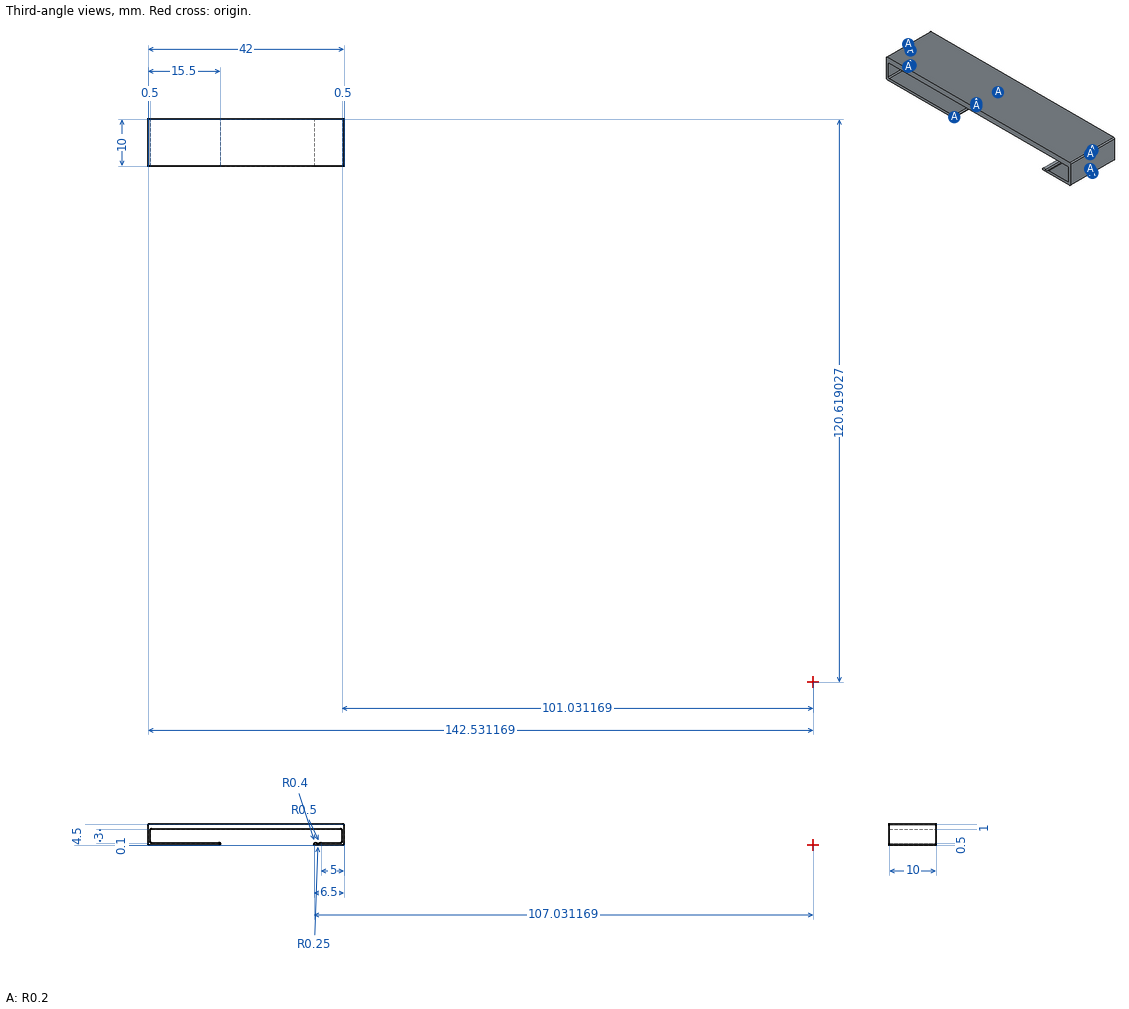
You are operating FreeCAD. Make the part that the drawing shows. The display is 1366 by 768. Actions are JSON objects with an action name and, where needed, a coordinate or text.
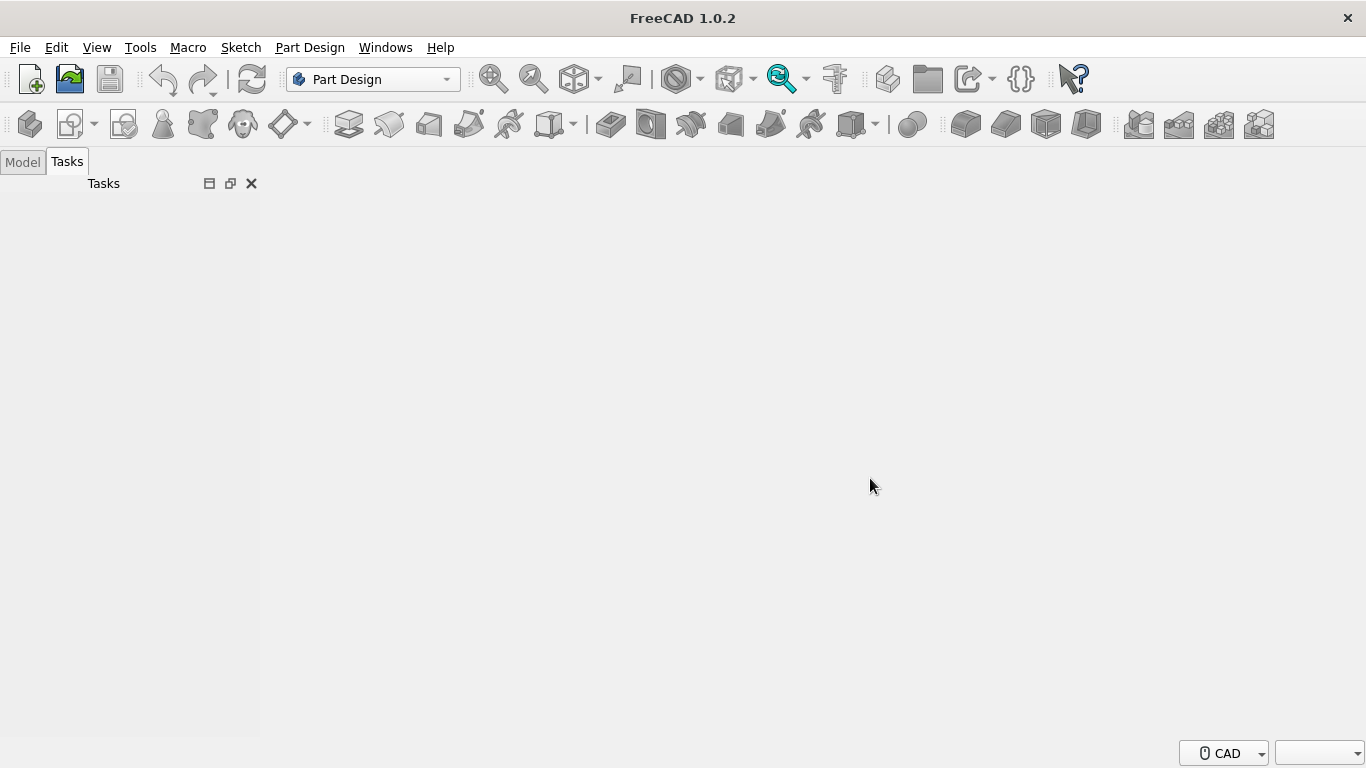
{"action": "left_click", "coordinate": [30, 80]}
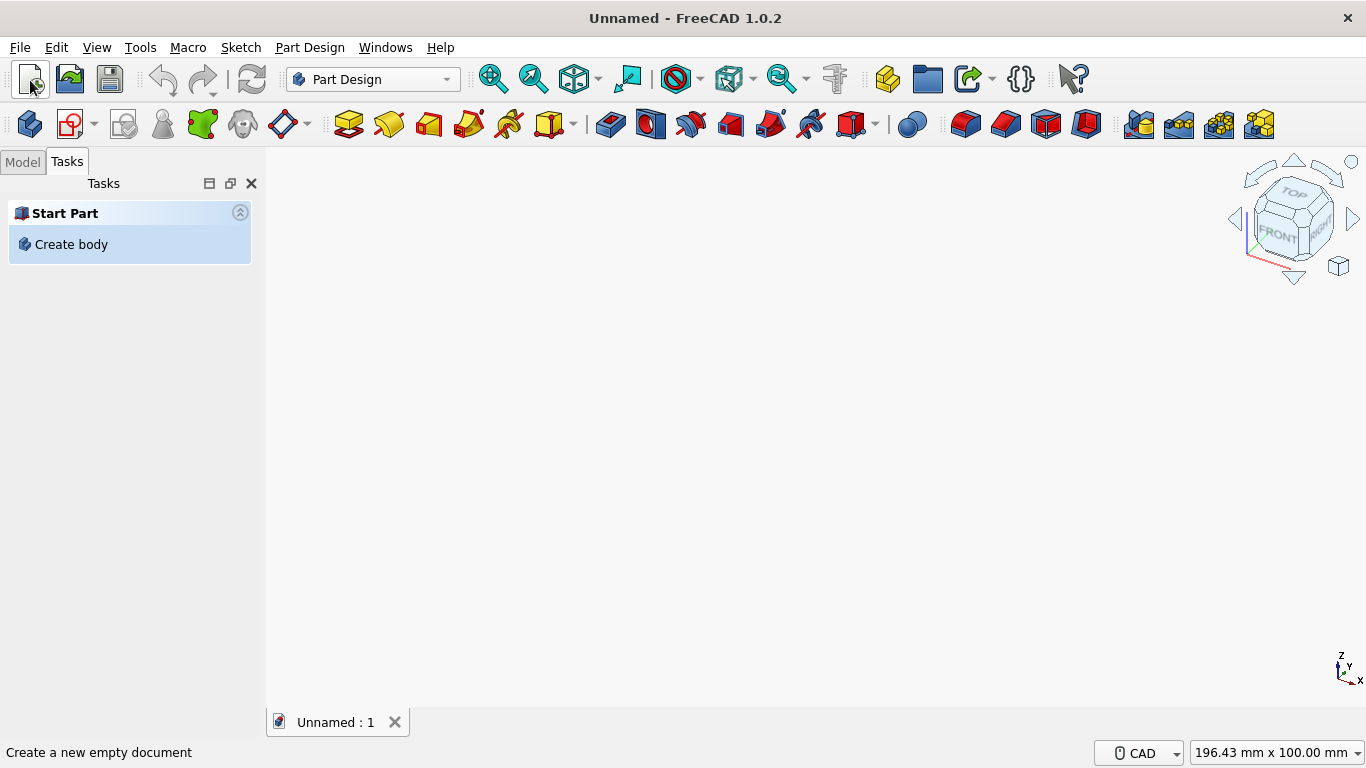
{"action": "left_click", "coordinate": [70, 124]}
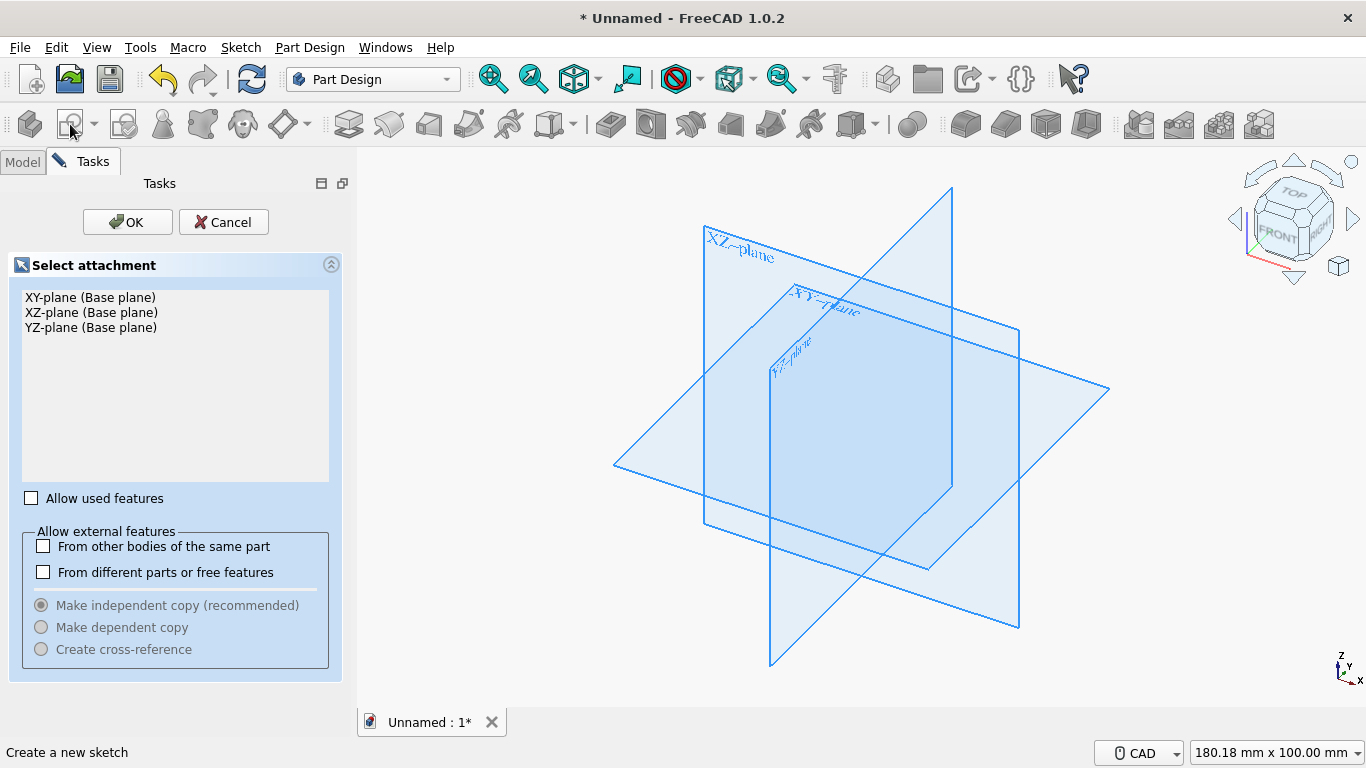
{"action": "left_click", "coordinate": [82, 298]}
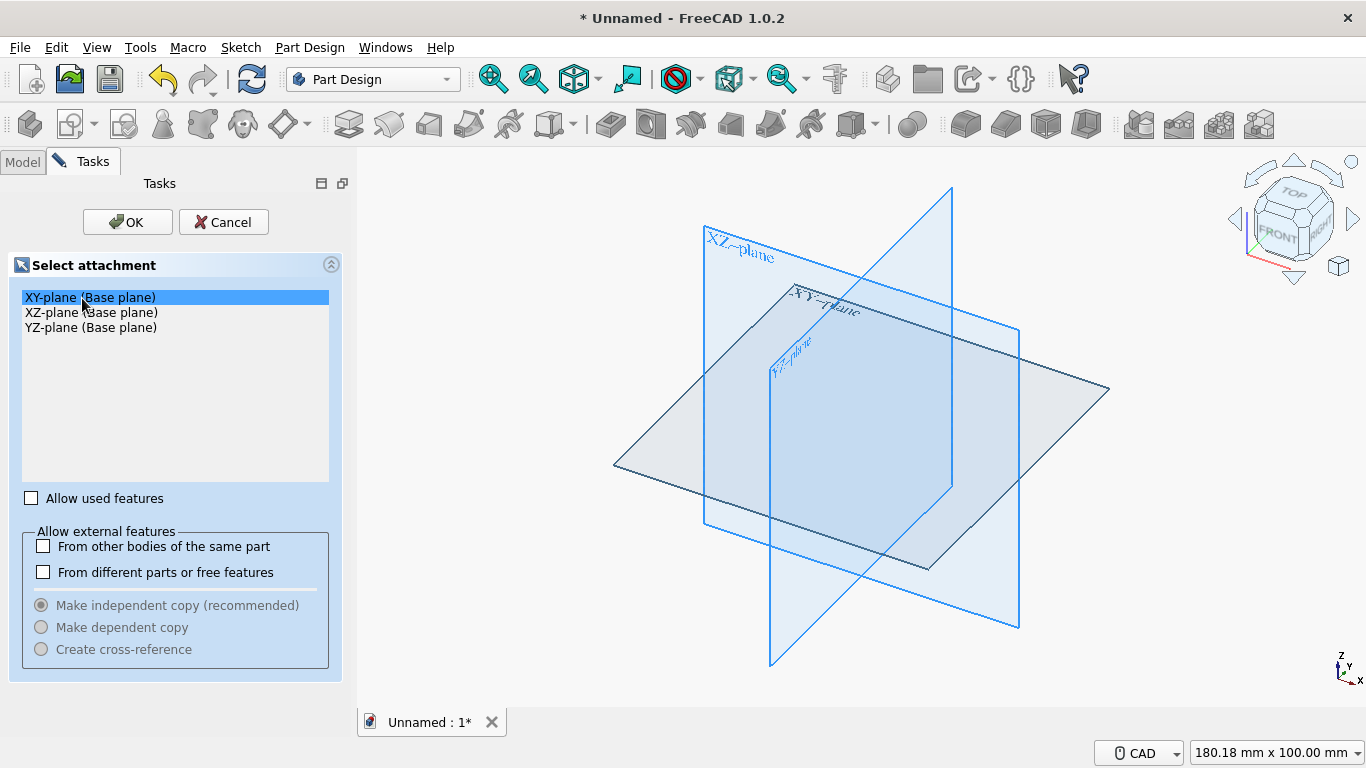
{"action": "left_click", "coordinate": [128, 222]}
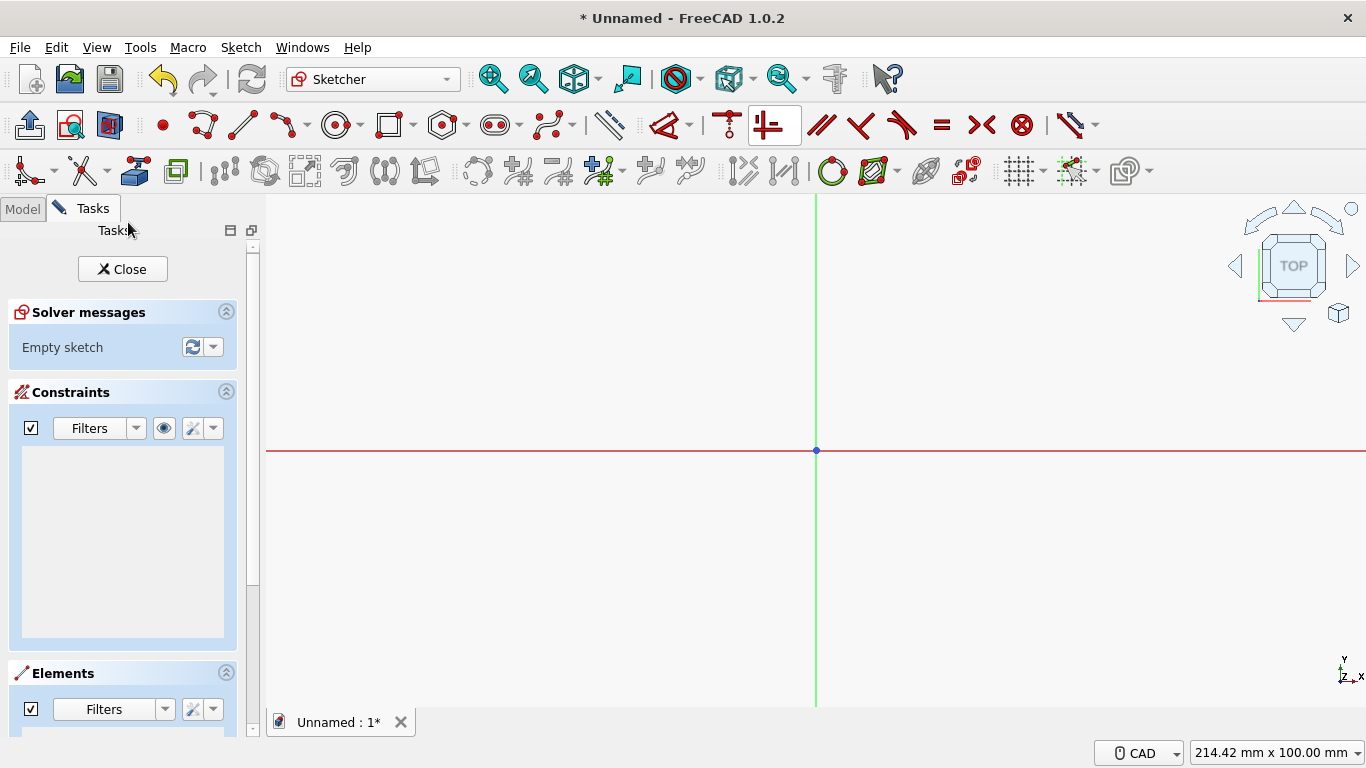
{"action": "scroll", "coordinate": [748, 450], "scroll_direction": "down", "scroll_amount": 5}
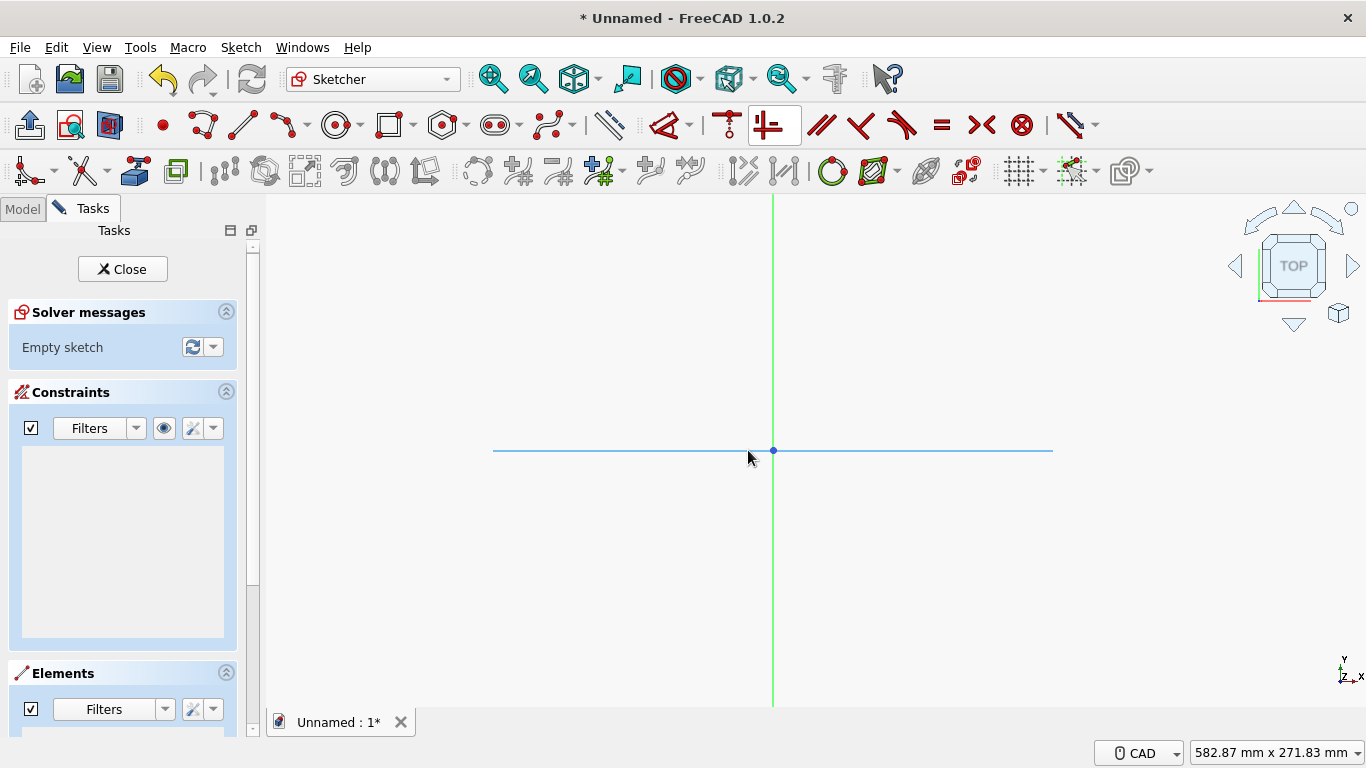
{"action": "scroll", "coordinate": [748, 450], "scroll_direction": "down", "scroll_amount": 5}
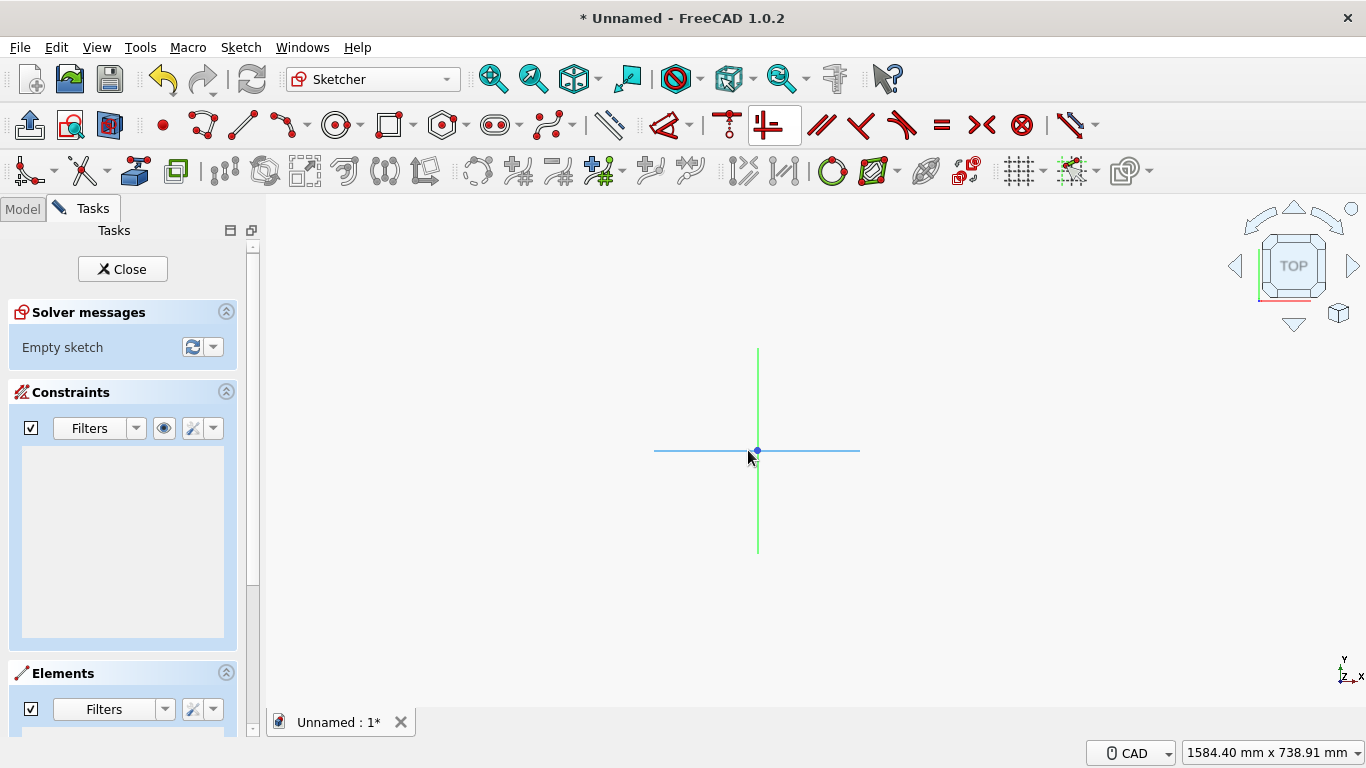
{"action": "scroll", "coordinate": [660, 366], "scroll_direction": "up", "scroll_amount": 15}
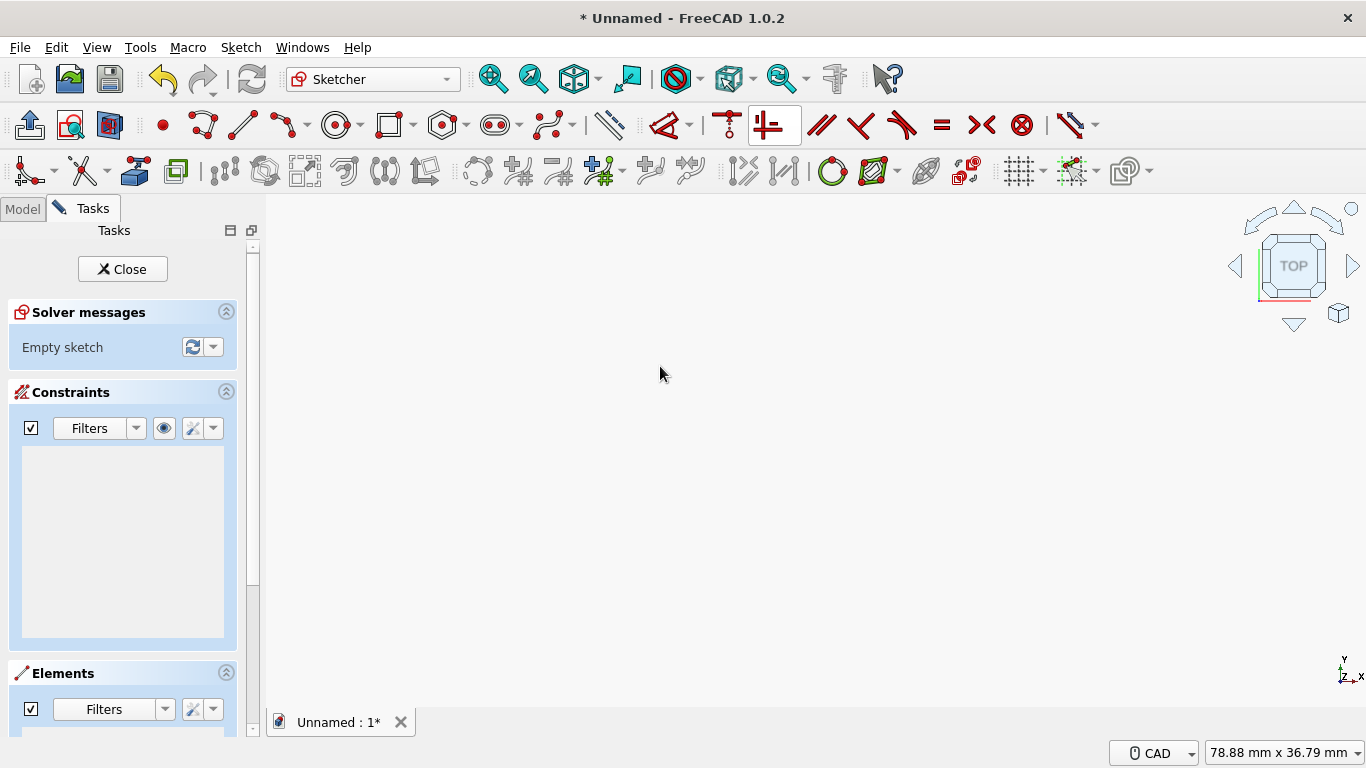
{"action": "scroll", "coordinate": [722, 440], "scroll_direction": "up", "scroll_amount": 4}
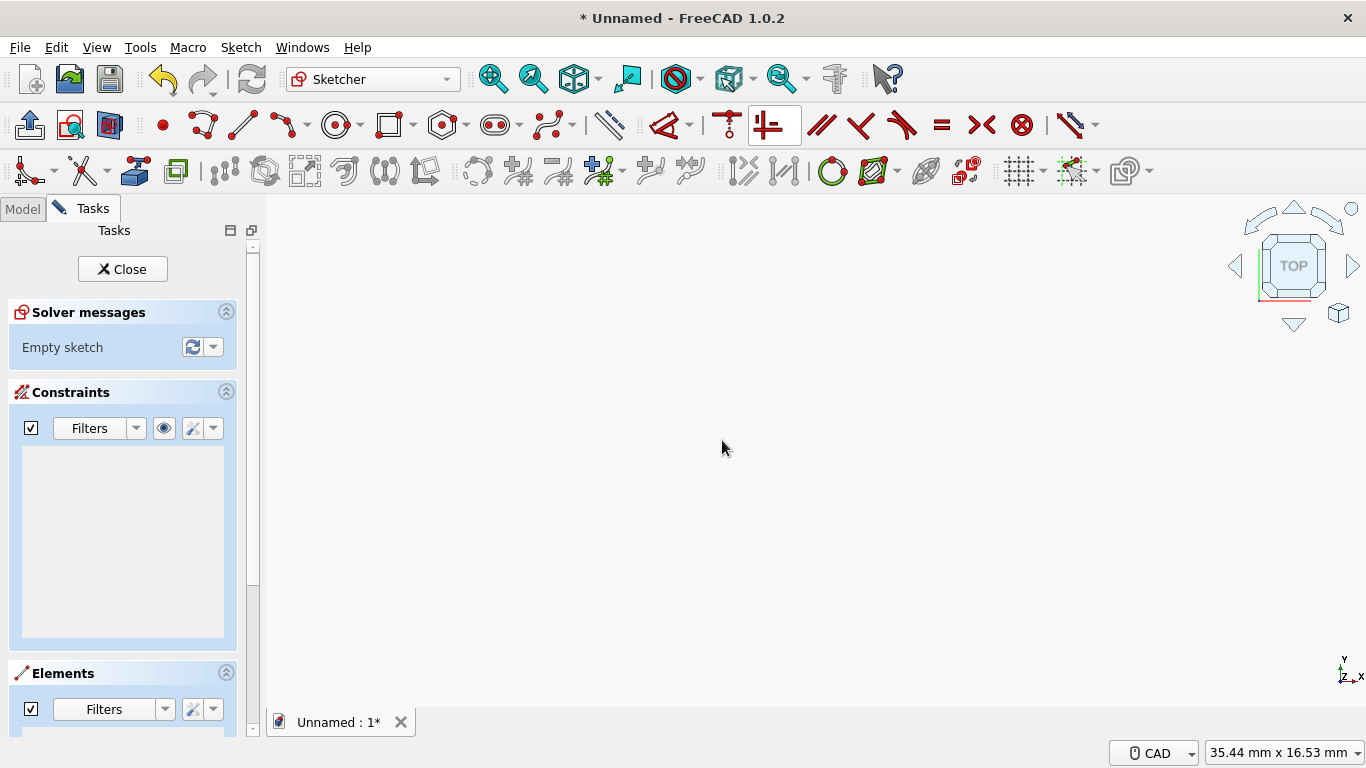
{"action": "left_click", "coordinate": [390, 126]}